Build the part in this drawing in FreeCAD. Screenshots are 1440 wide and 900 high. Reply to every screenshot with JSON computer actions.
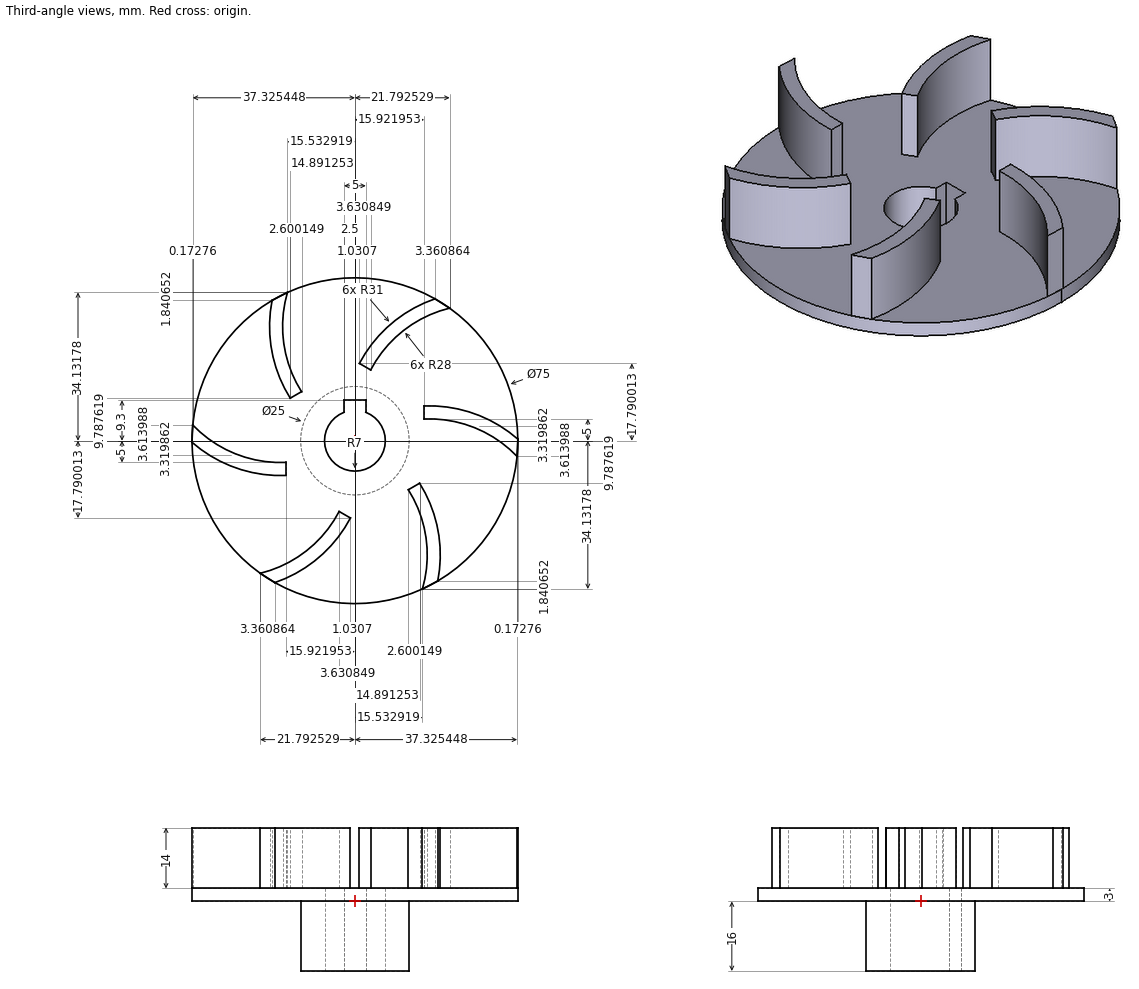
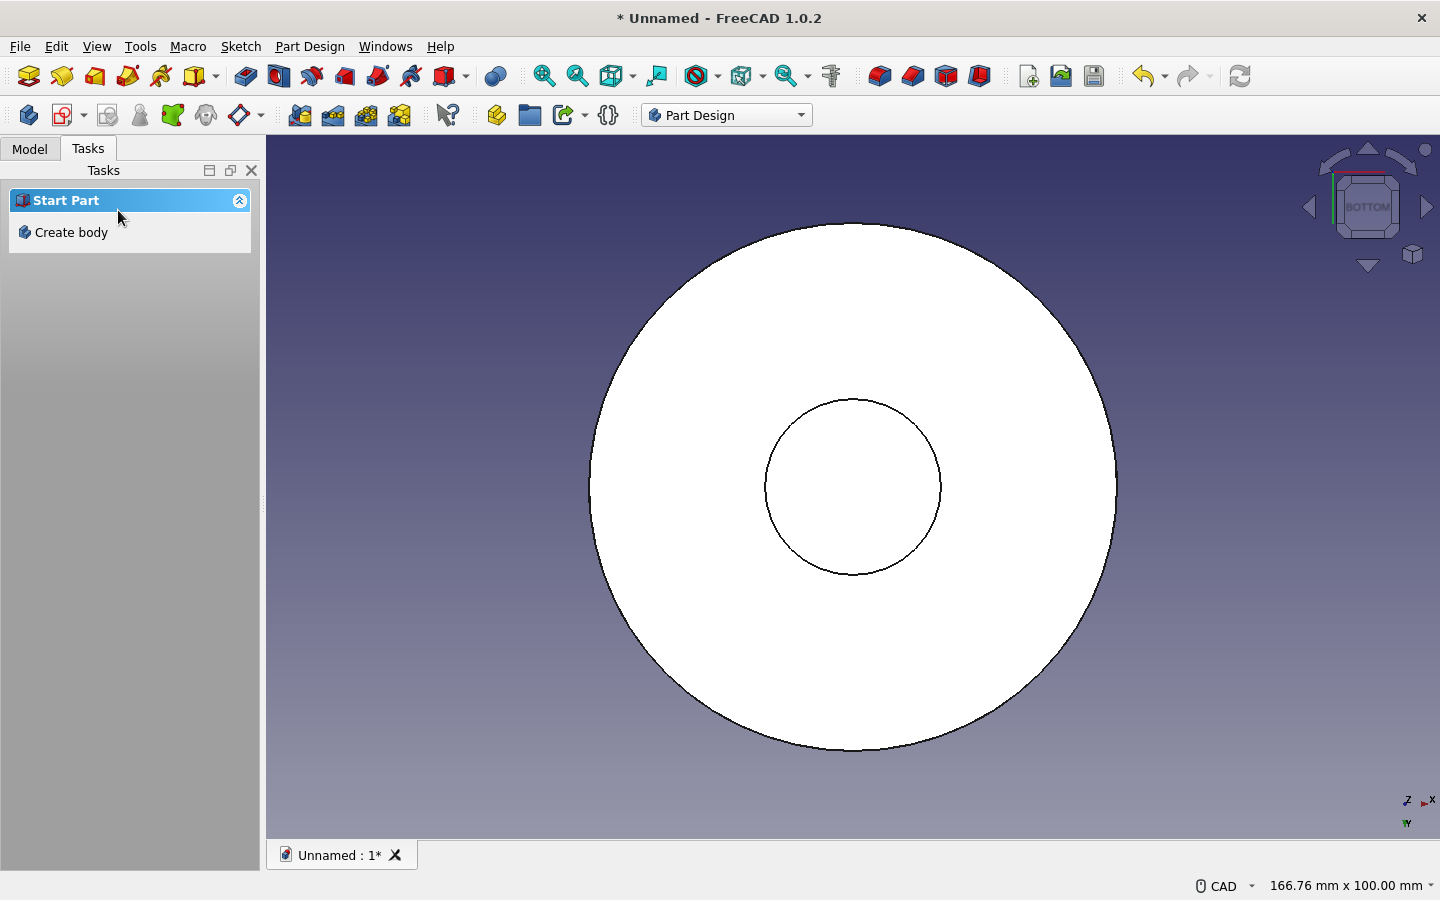
{"action": "left_click", "coordinate": [853, 486]}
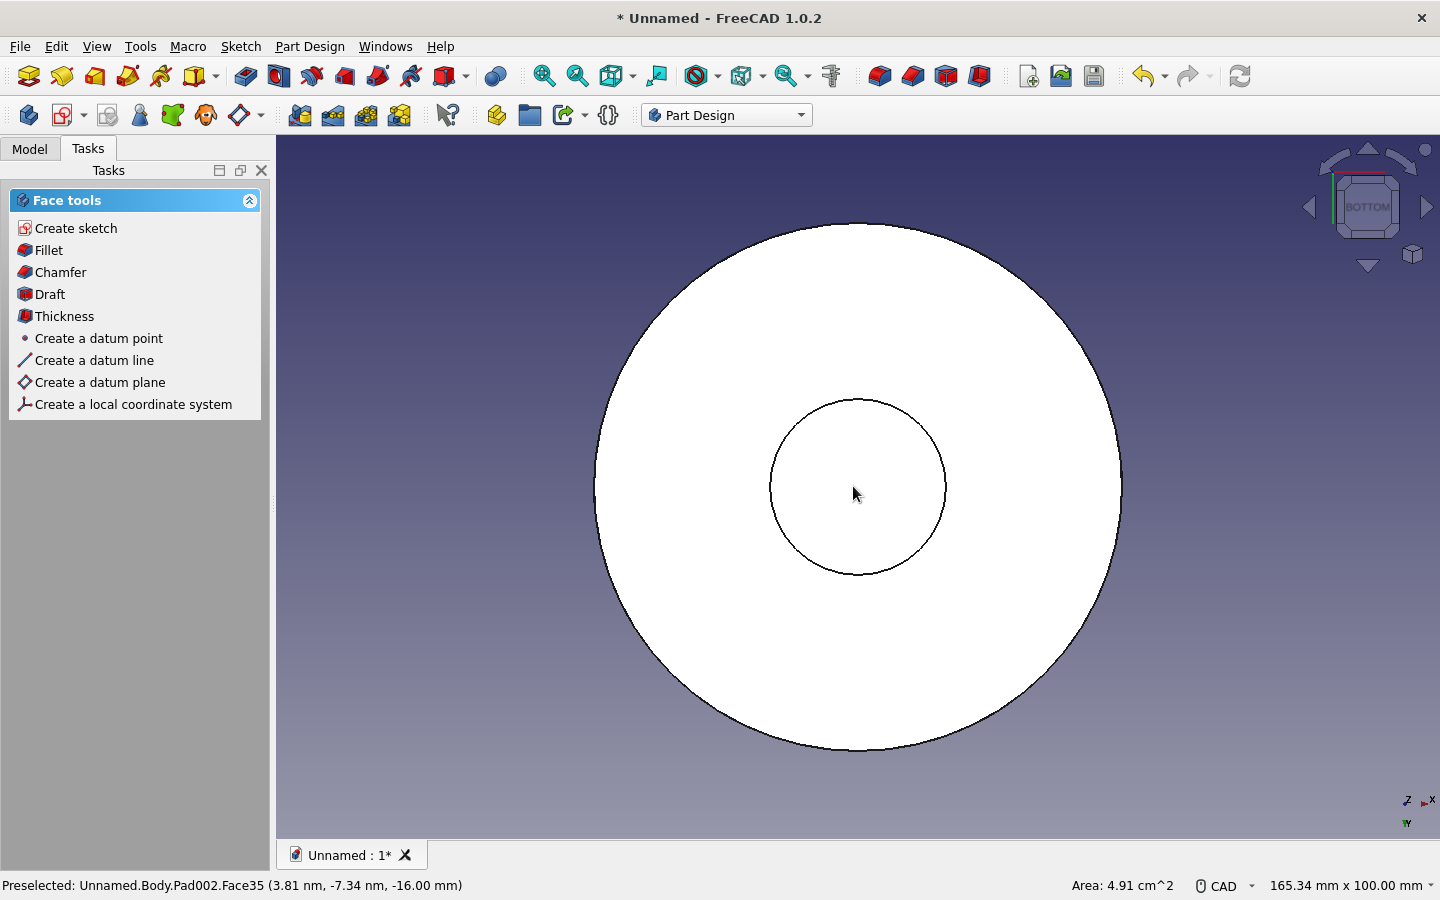
{"action": "left_click", "coordinate": [62, 116]}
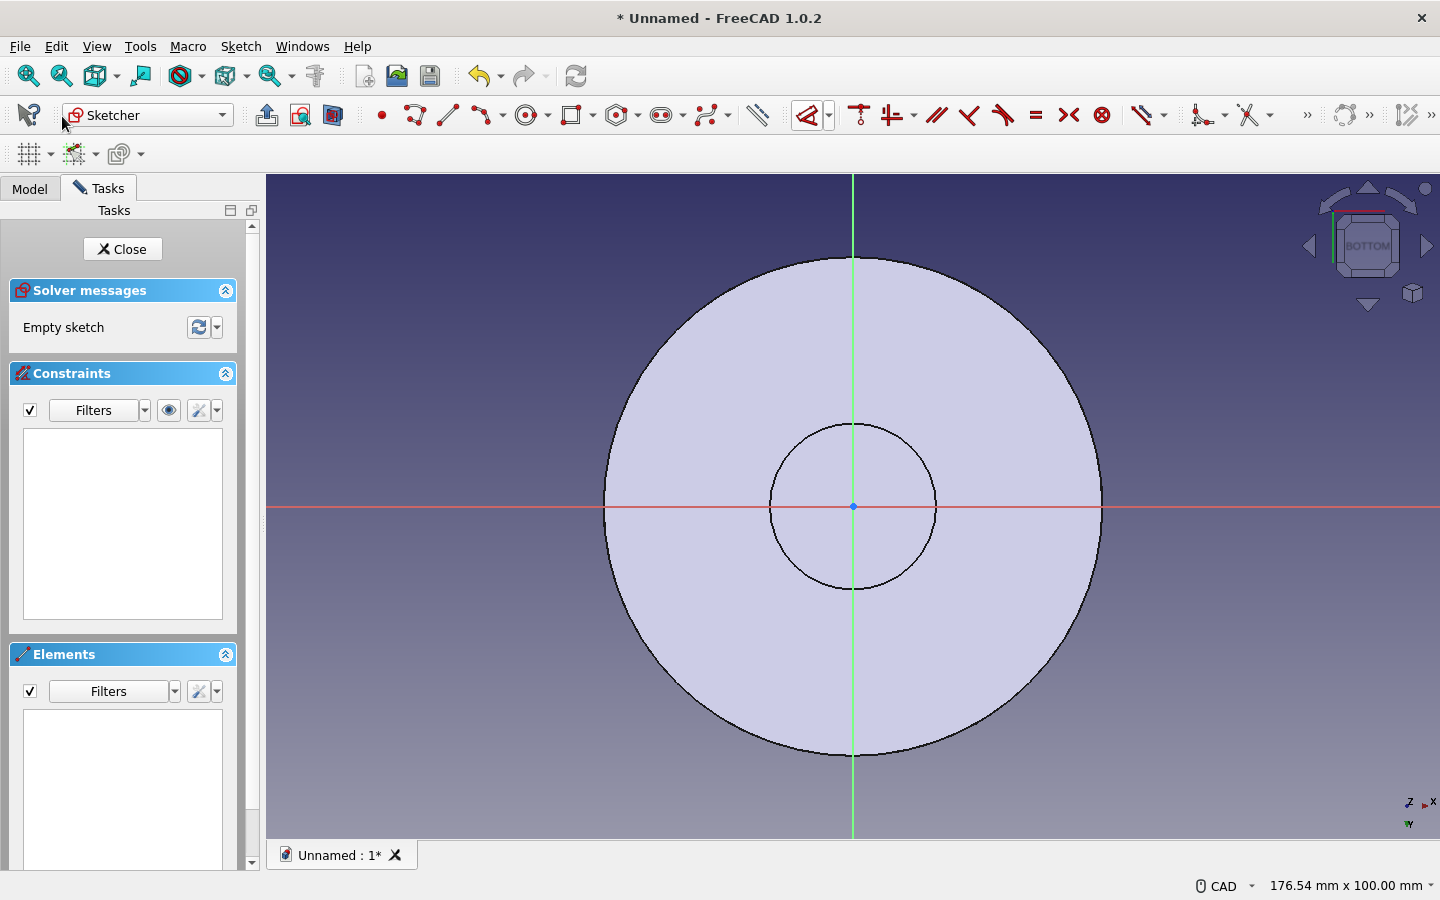
{"action": "scroll", "coordinate": [875, 517], "scroll_direction": "up", "scroll_amount": 7}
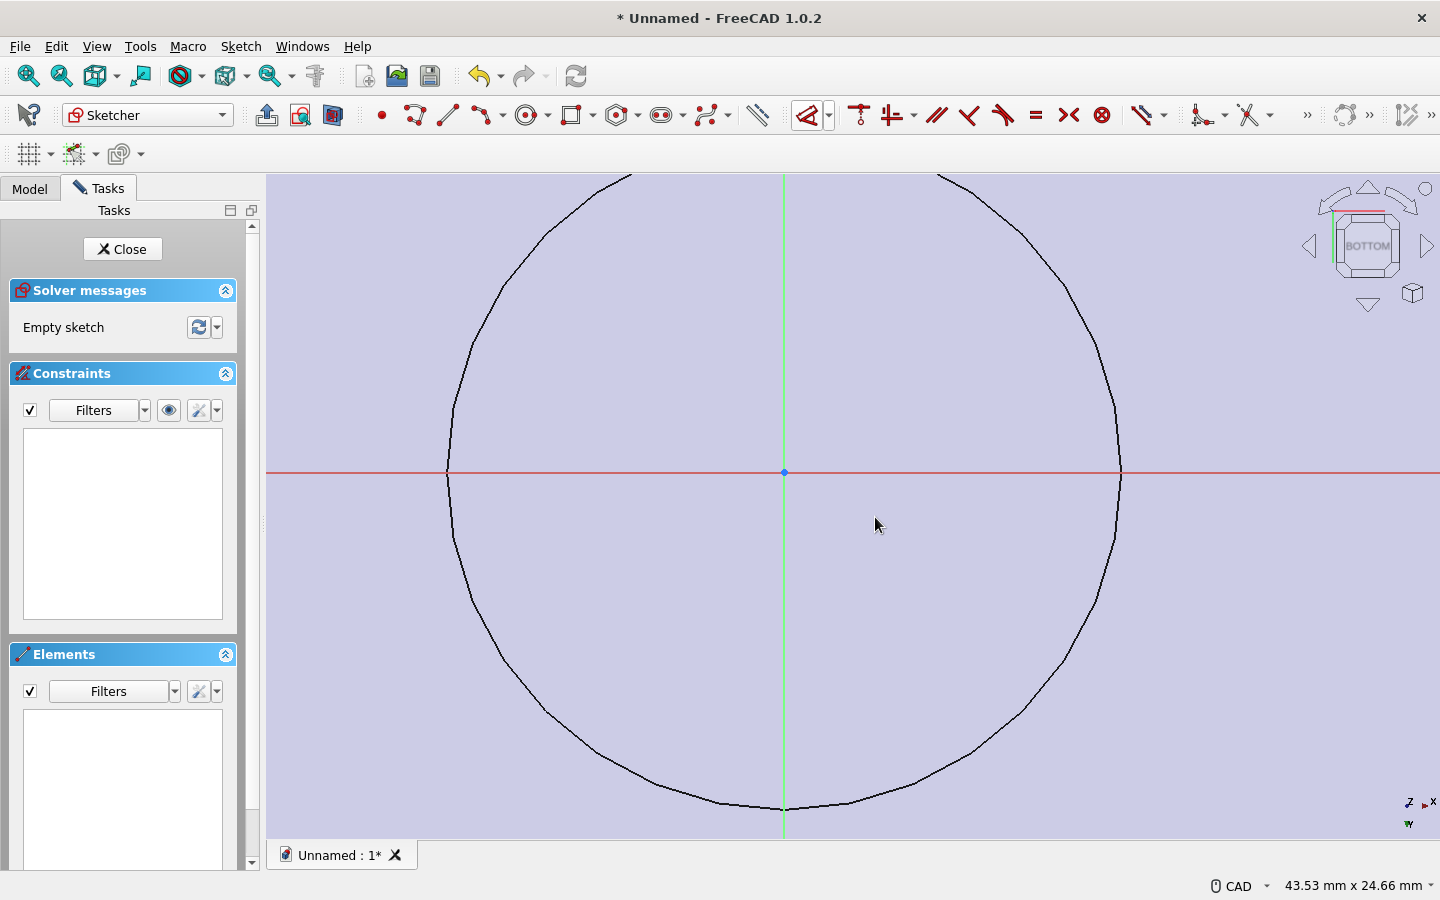
{"action": "left_click", "coordinate": [415, 116]}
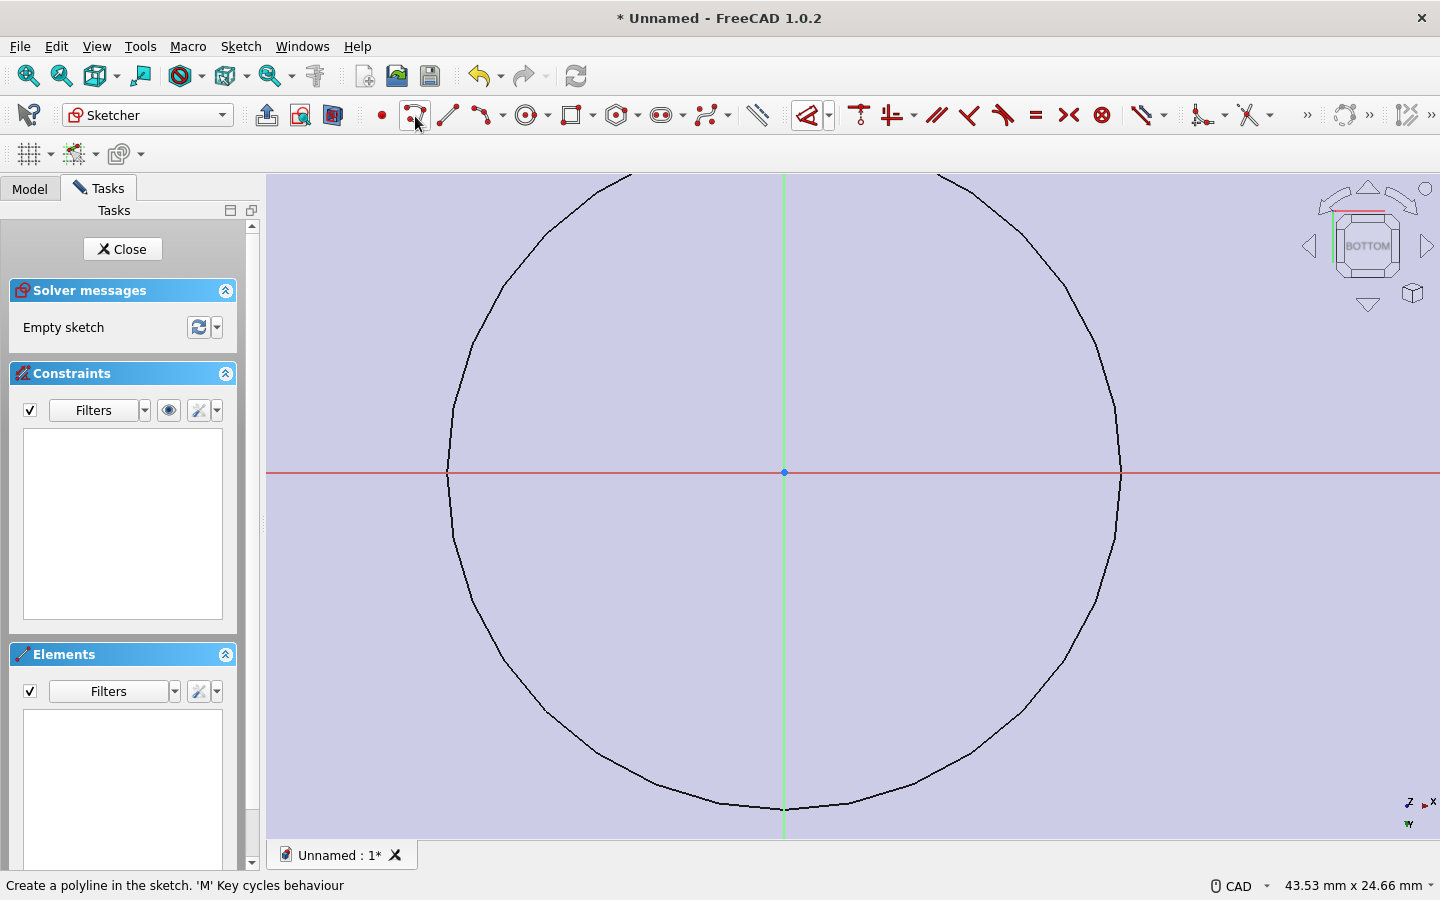
{"action": "left_click", "coordinate": [717, 649]}
{"action": "left_click", "coordinate": [717, 724]}
{"action": "left_click", "coordinate": [852, 724]}
{"action": "left_click", "coordinate": [852, 649]}
{"action": "right_click", "coordinate": [852, 649]}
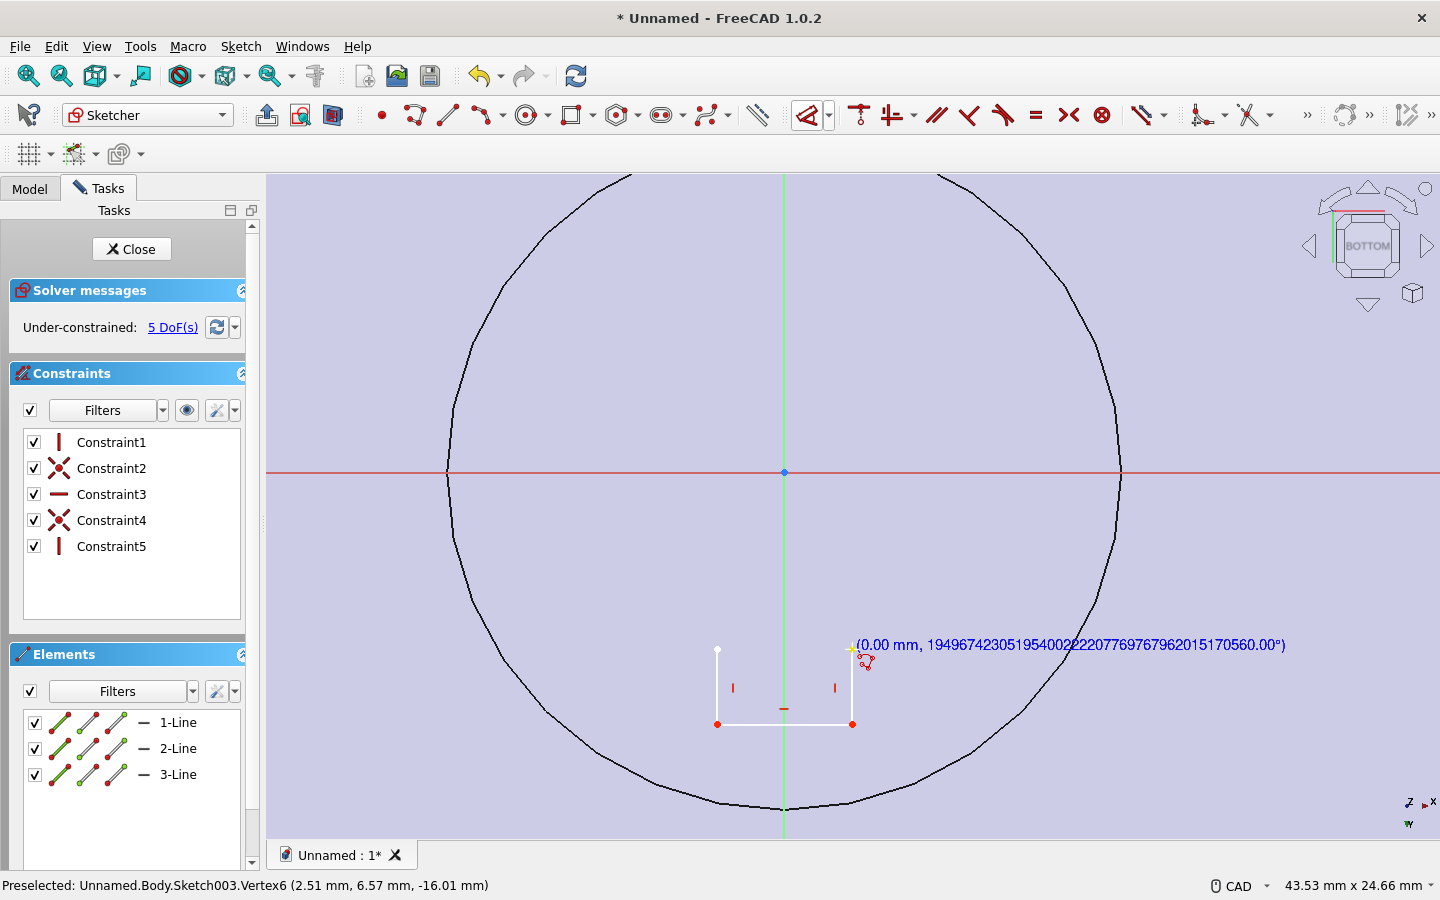
{"action": "key", "text": "g 3 a"}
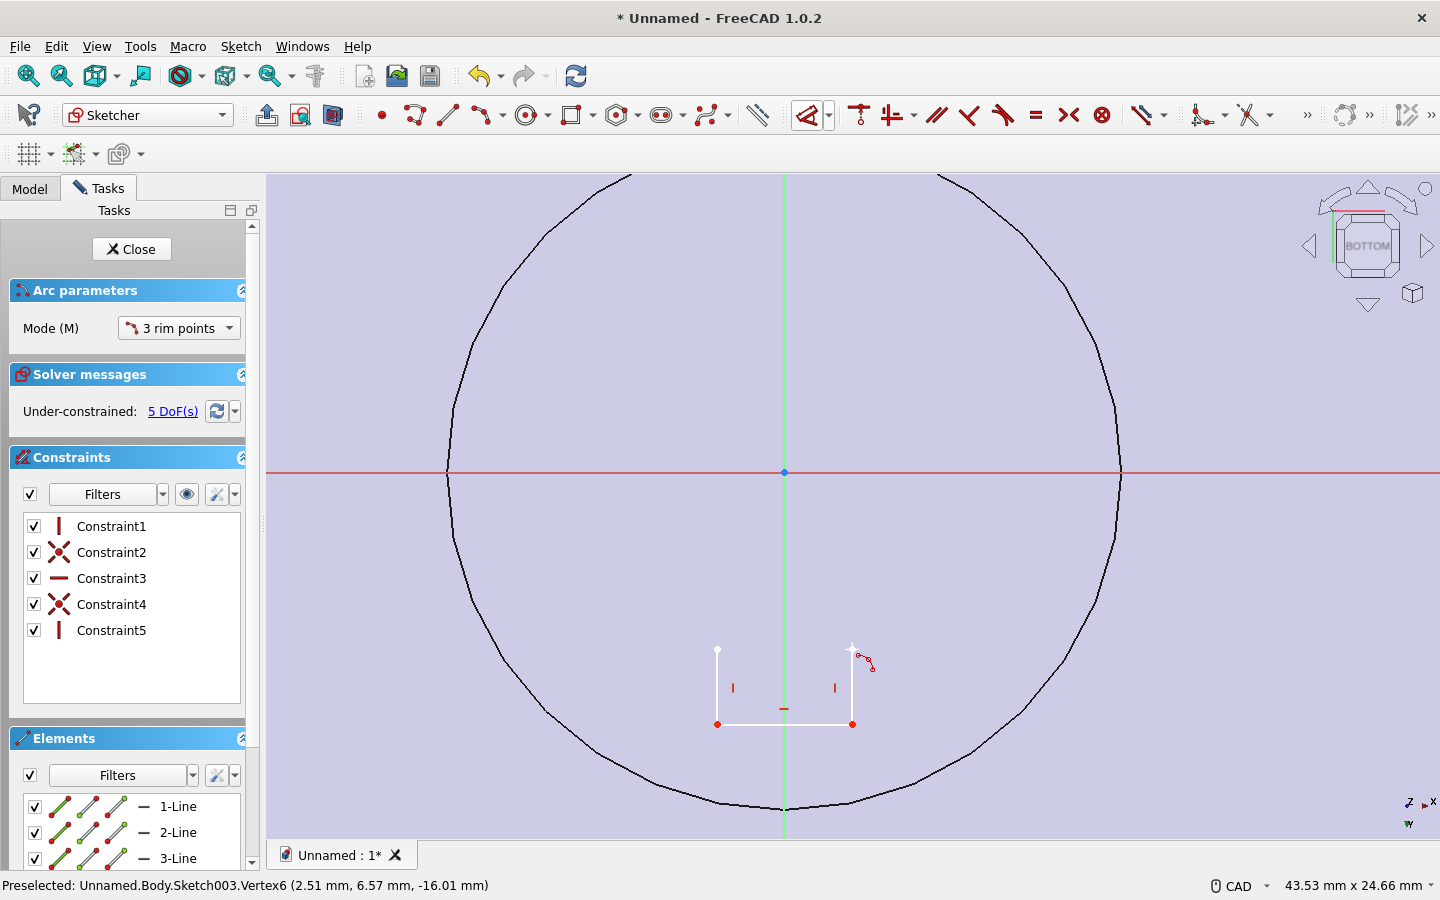
{"action": "left_click", "coordinate": [852, 650]}
{"action": "left_click", "coordinate": [717, 650]}
{"action": "left_click", "coordinate": [884, 312]}
{"action": "key", "text": "Escape"}